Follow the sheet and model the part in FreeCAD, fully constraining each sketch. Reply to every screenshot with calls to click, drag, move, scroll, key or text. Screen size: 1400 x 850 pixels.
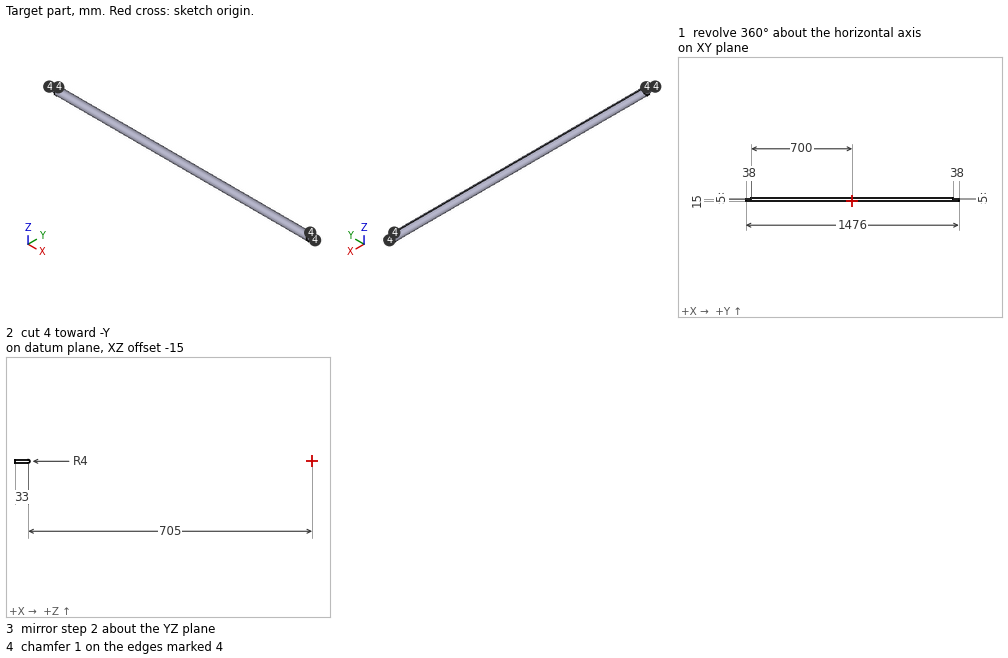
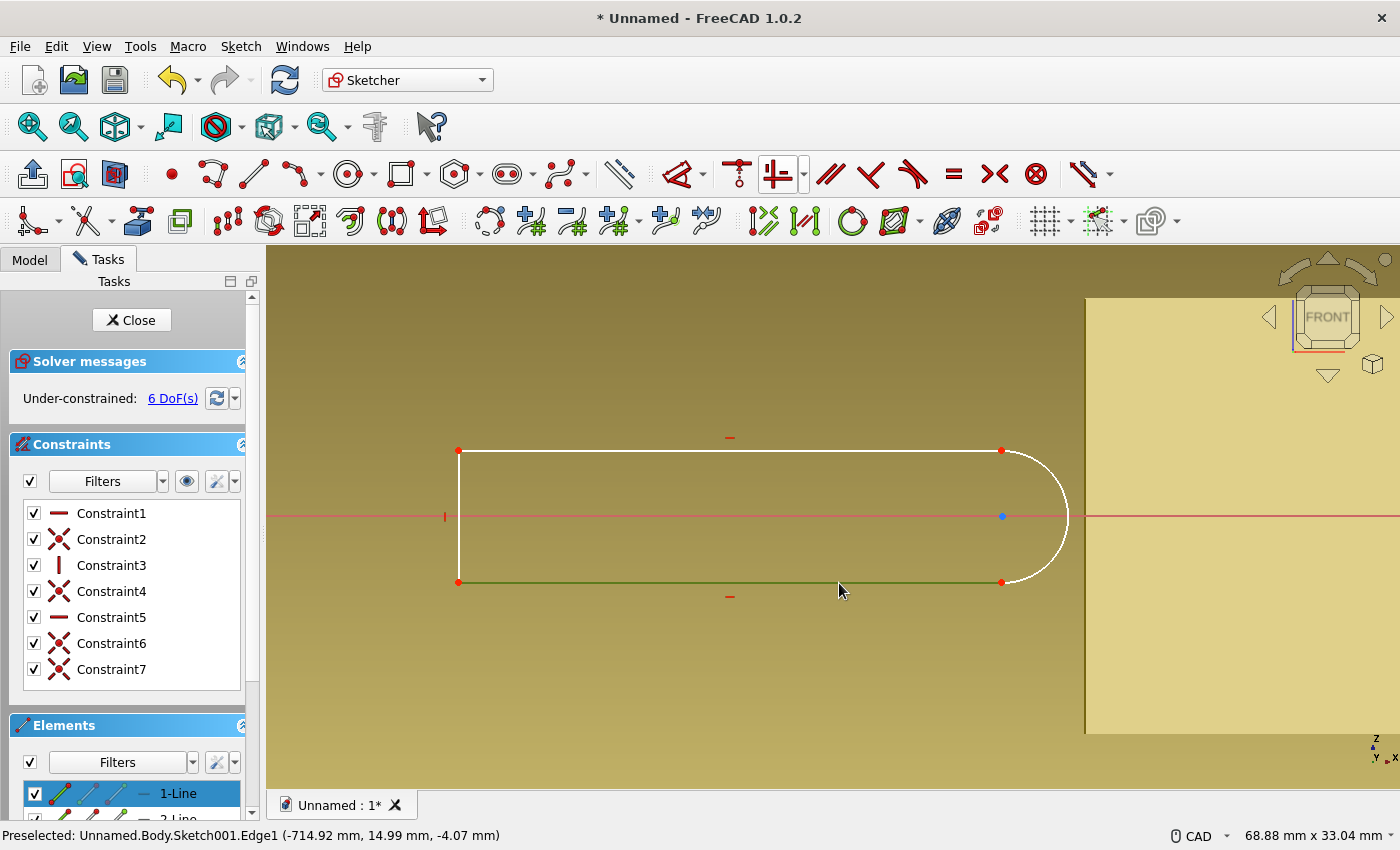
click(1055, 556)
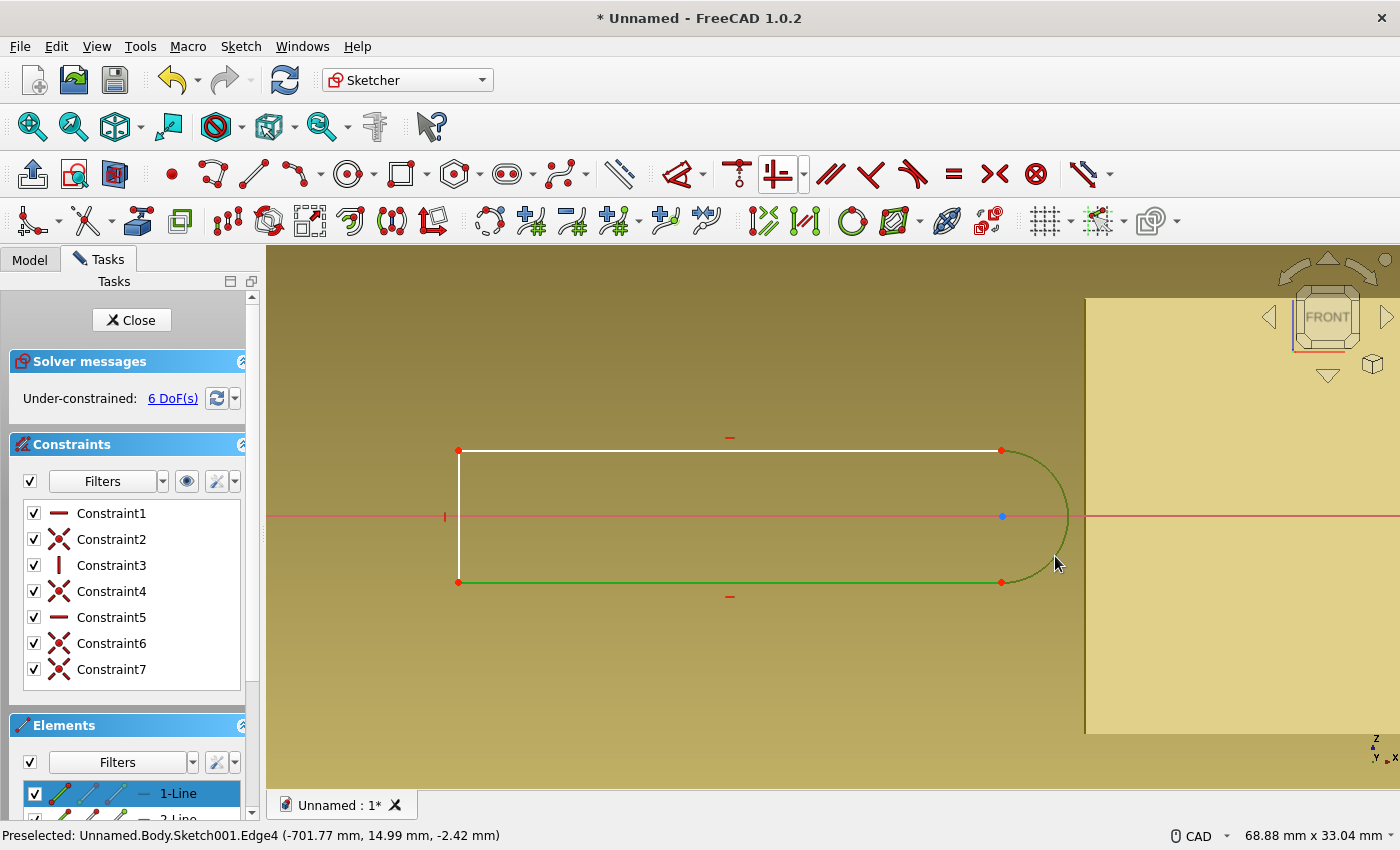
click(913, 174)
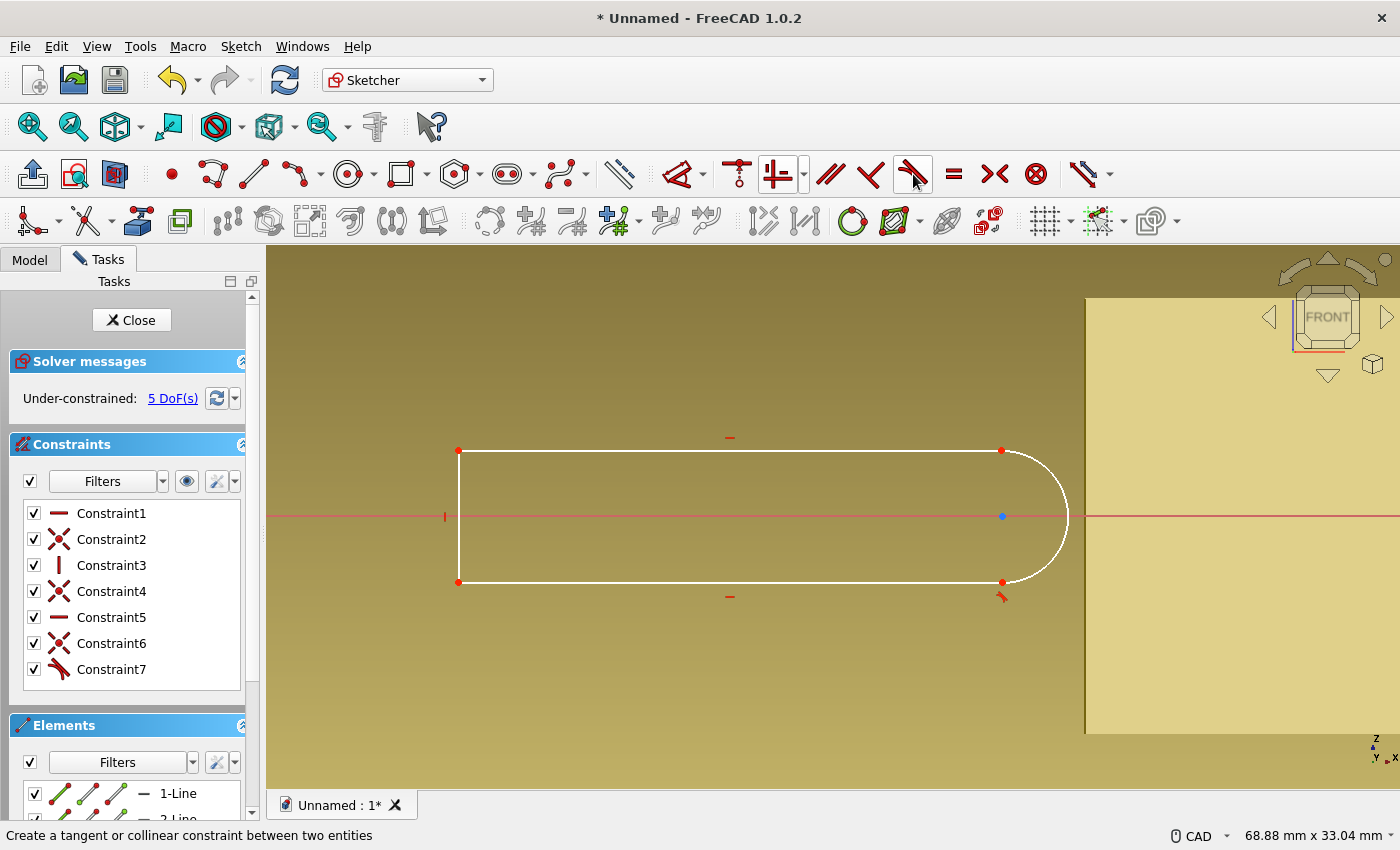
click(622, 451)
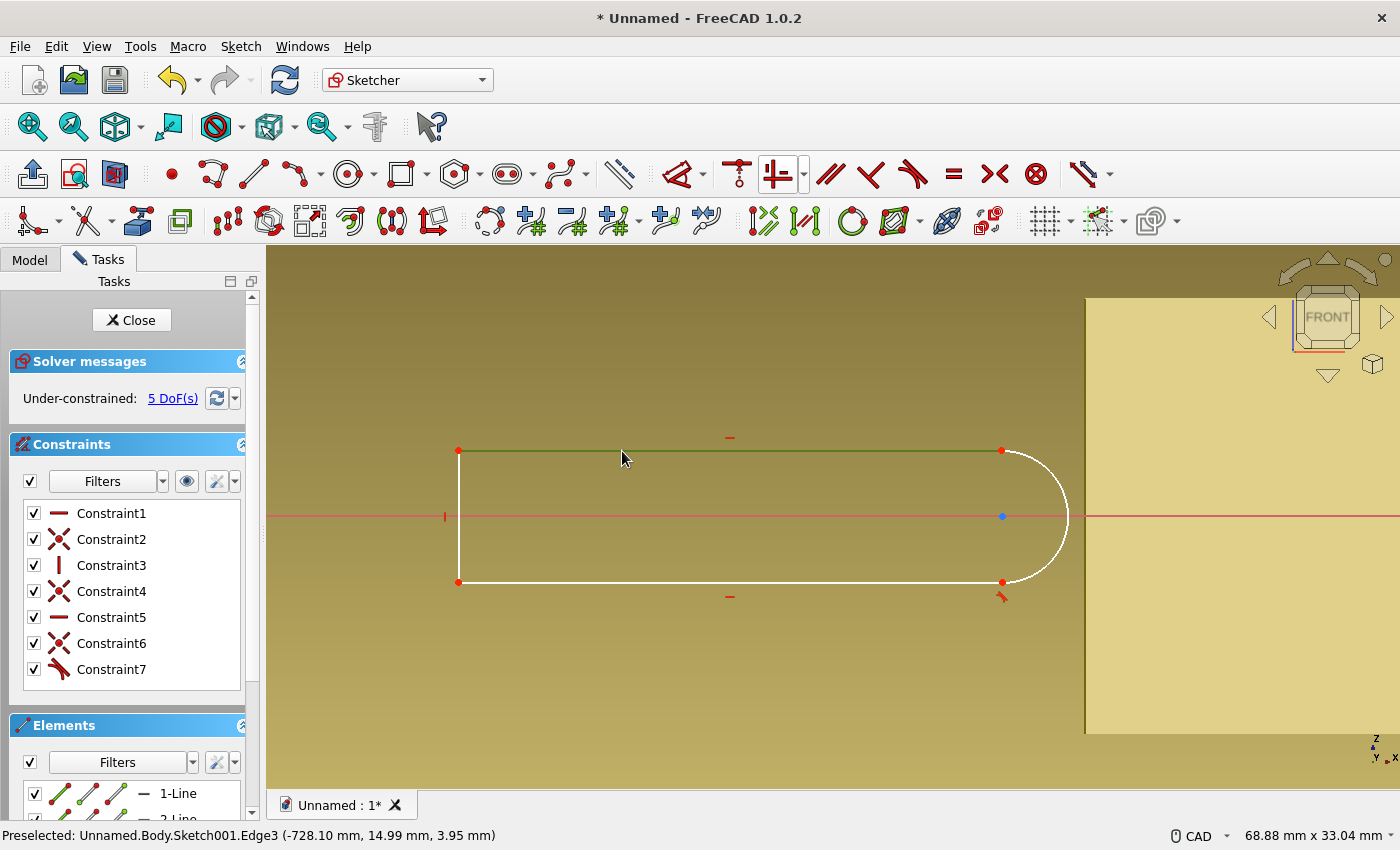
click(1056, 556)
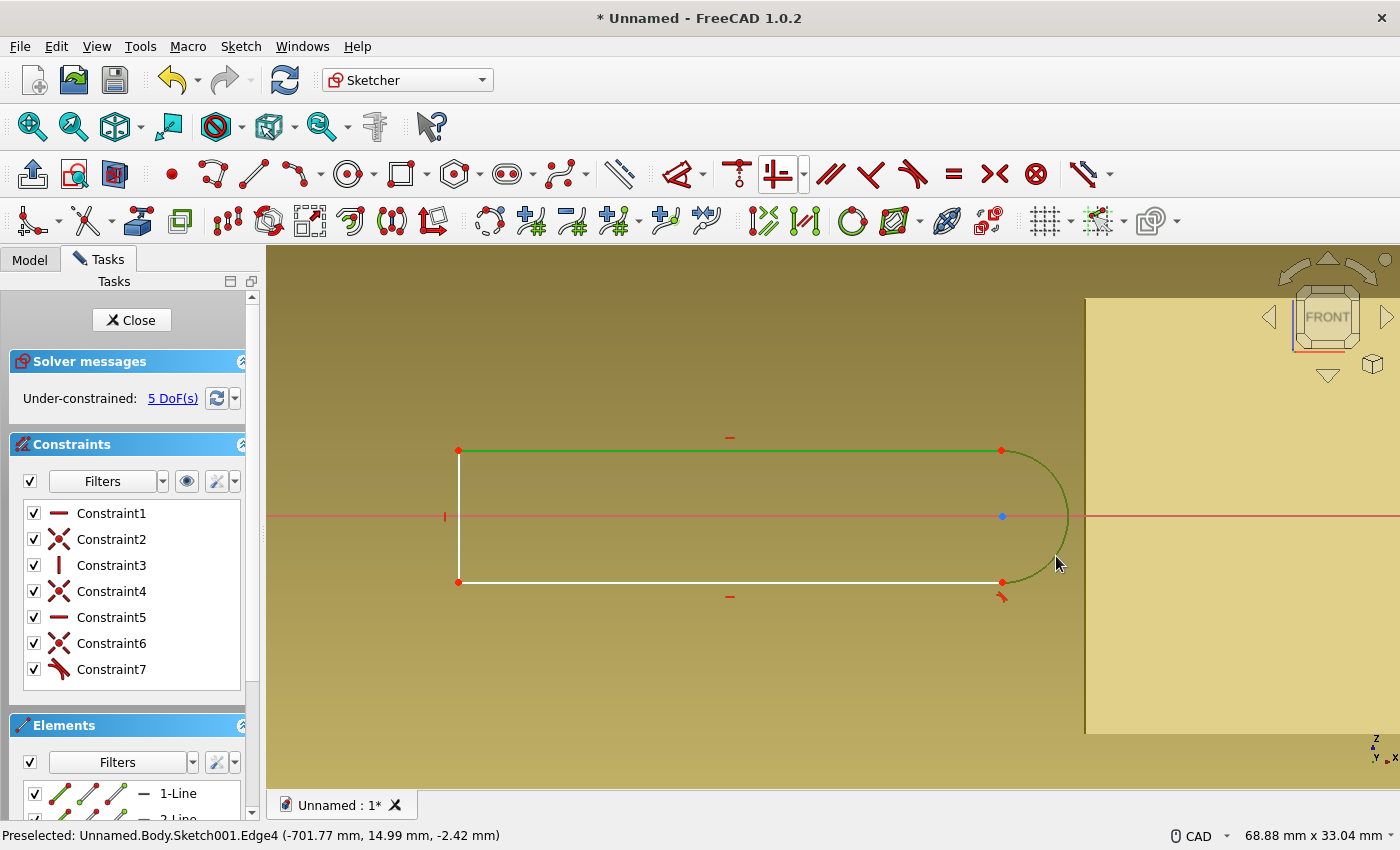
click(913, 174)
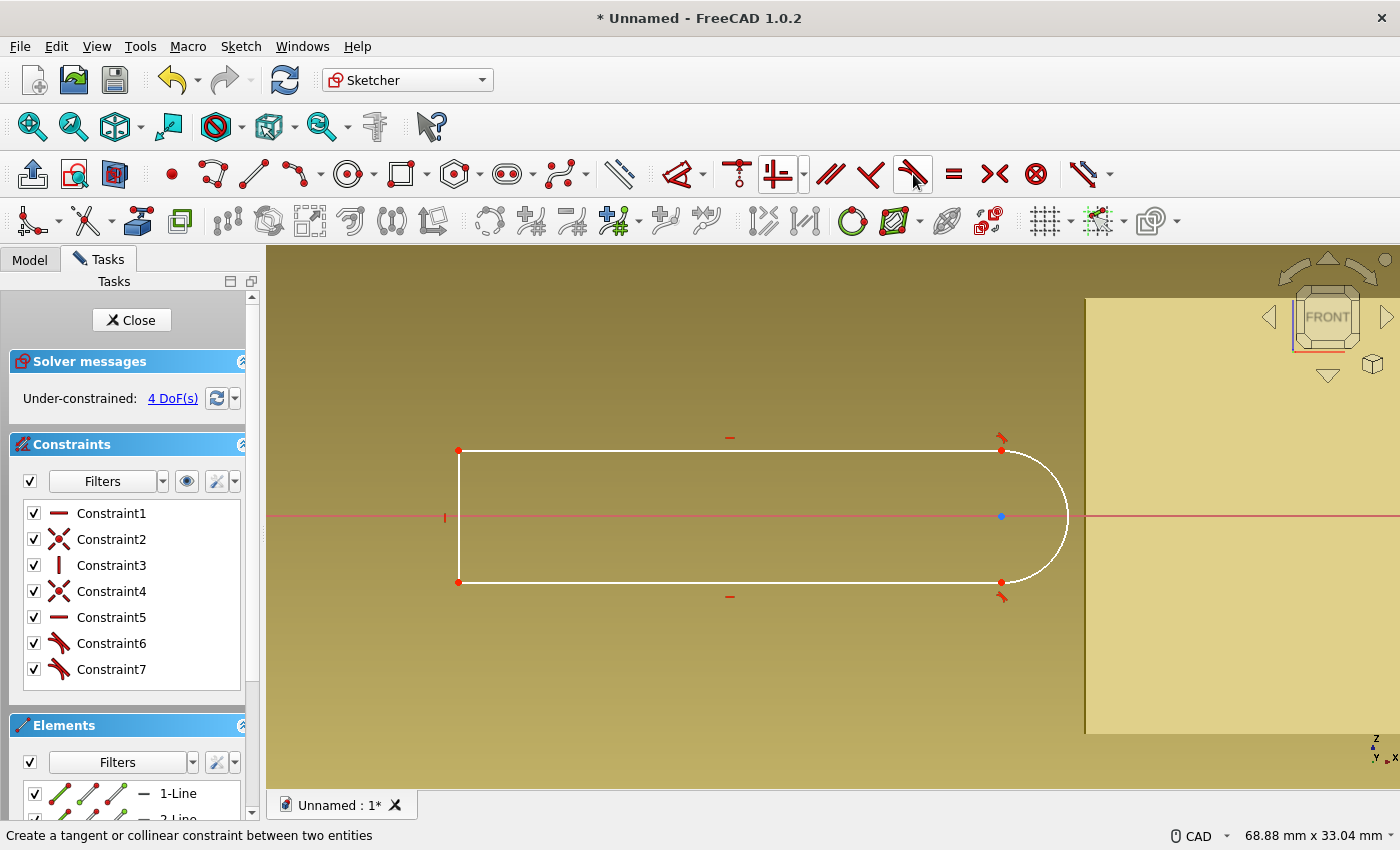
click(1002, 517)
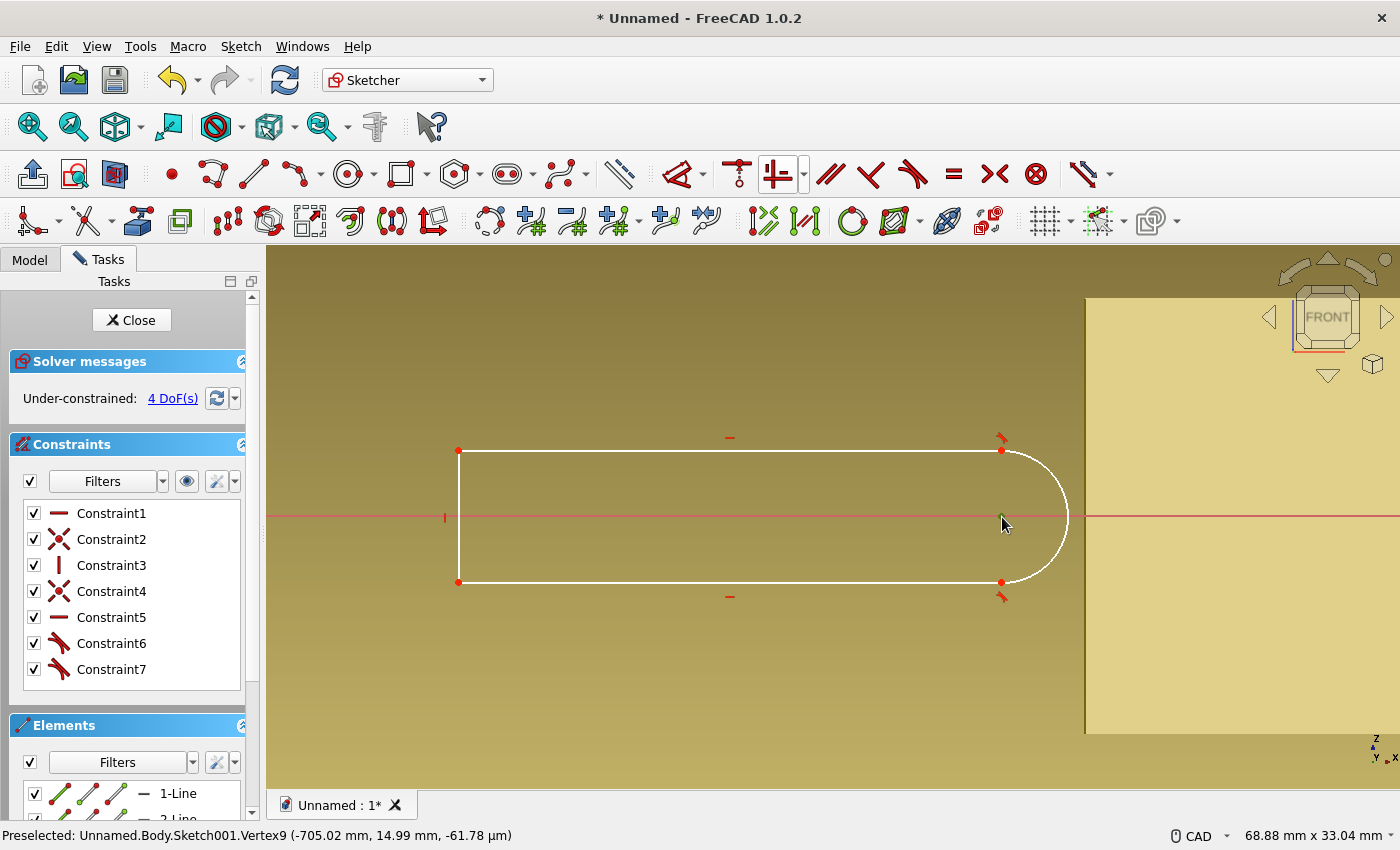
click(361, 516)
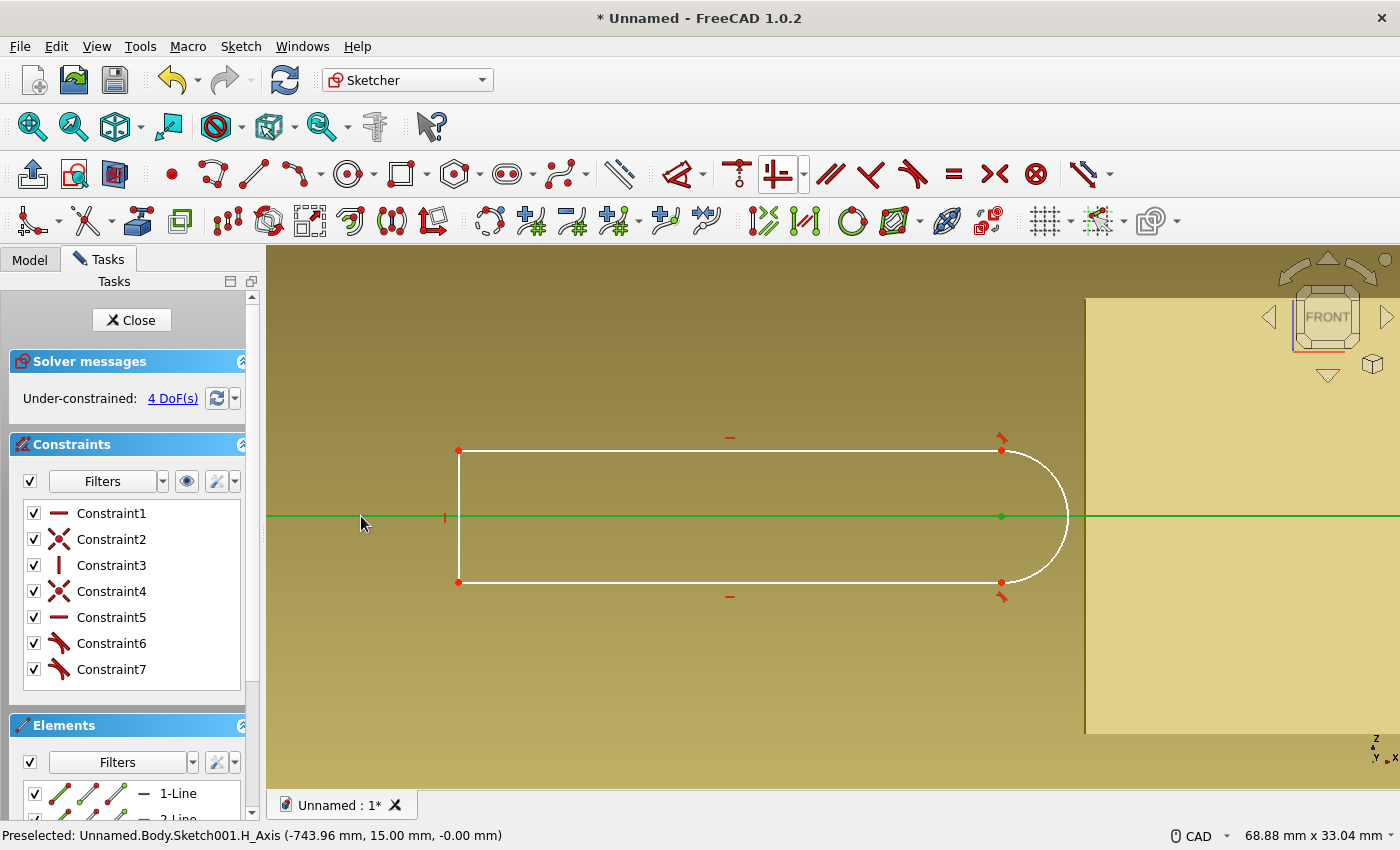
click(737, 174)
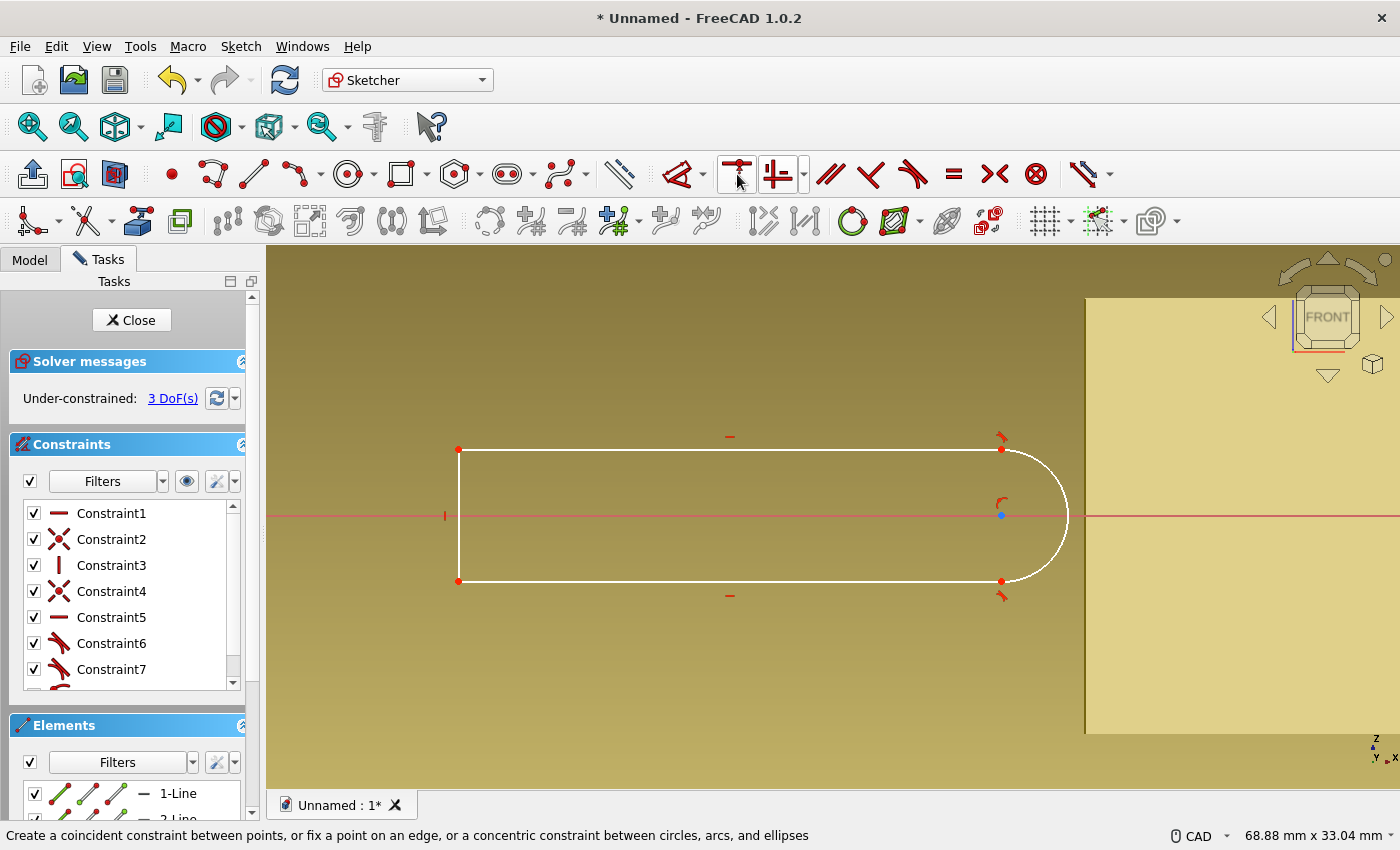
click(676, 174)